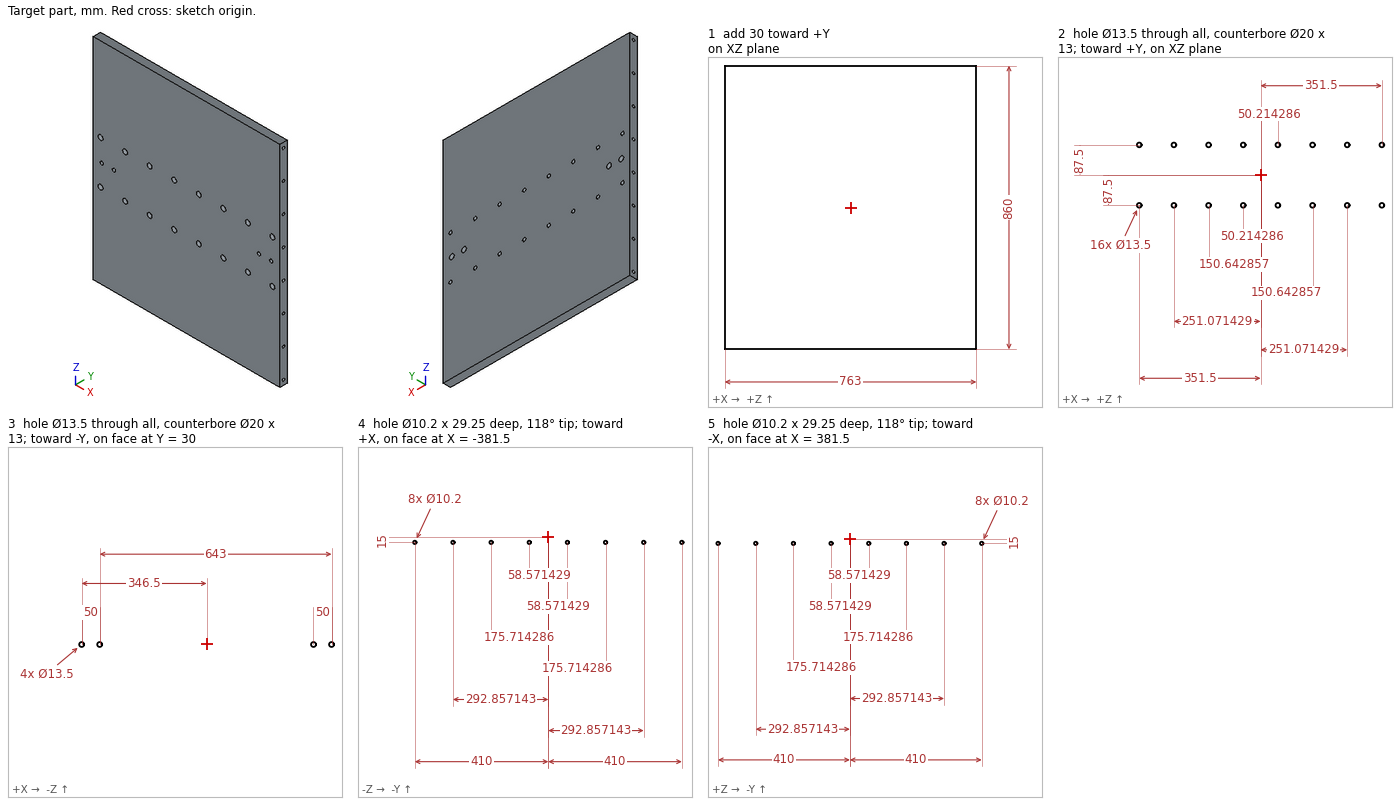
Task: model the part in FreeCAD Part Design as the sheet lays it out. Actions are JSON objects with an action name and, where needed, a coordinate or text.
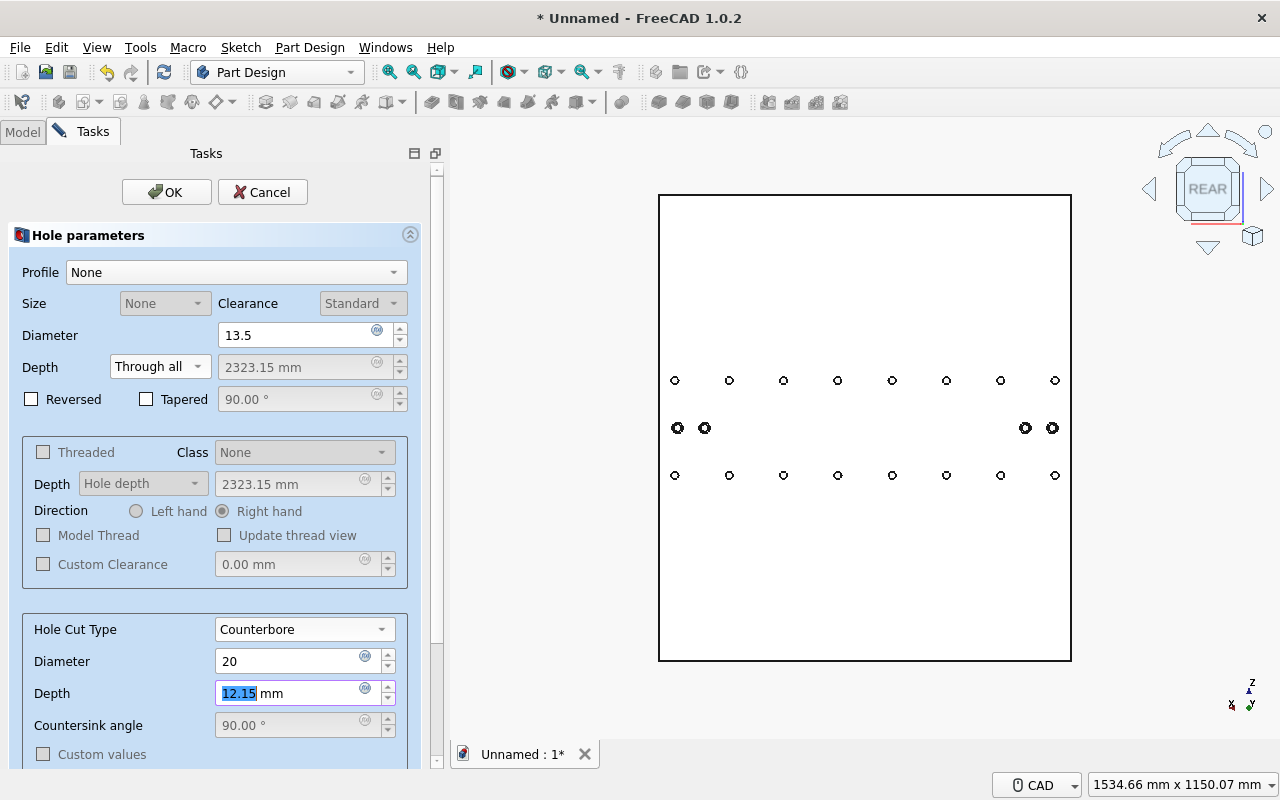
{"action": "type", "text": "13"}
{"action": "key", "text": "Tab"}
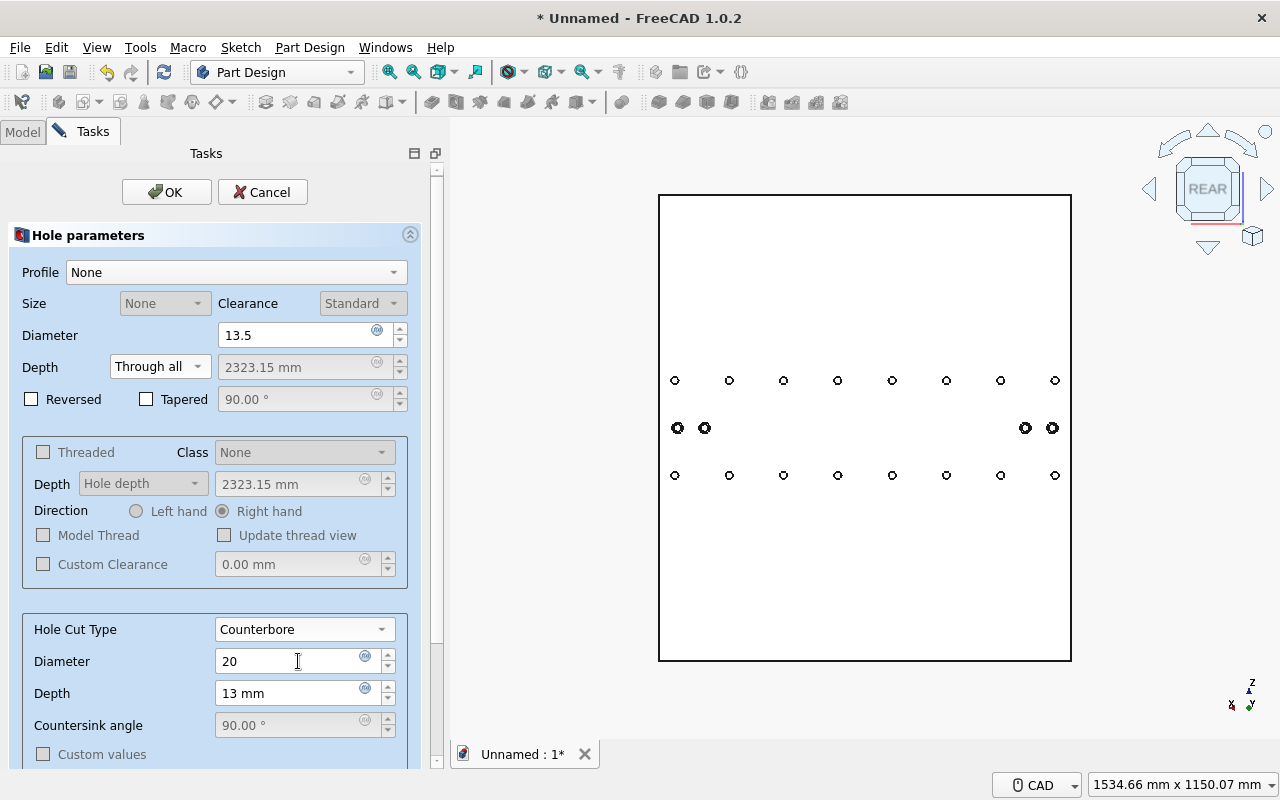
{"action": "left_click", "coordinate": [167, 192]}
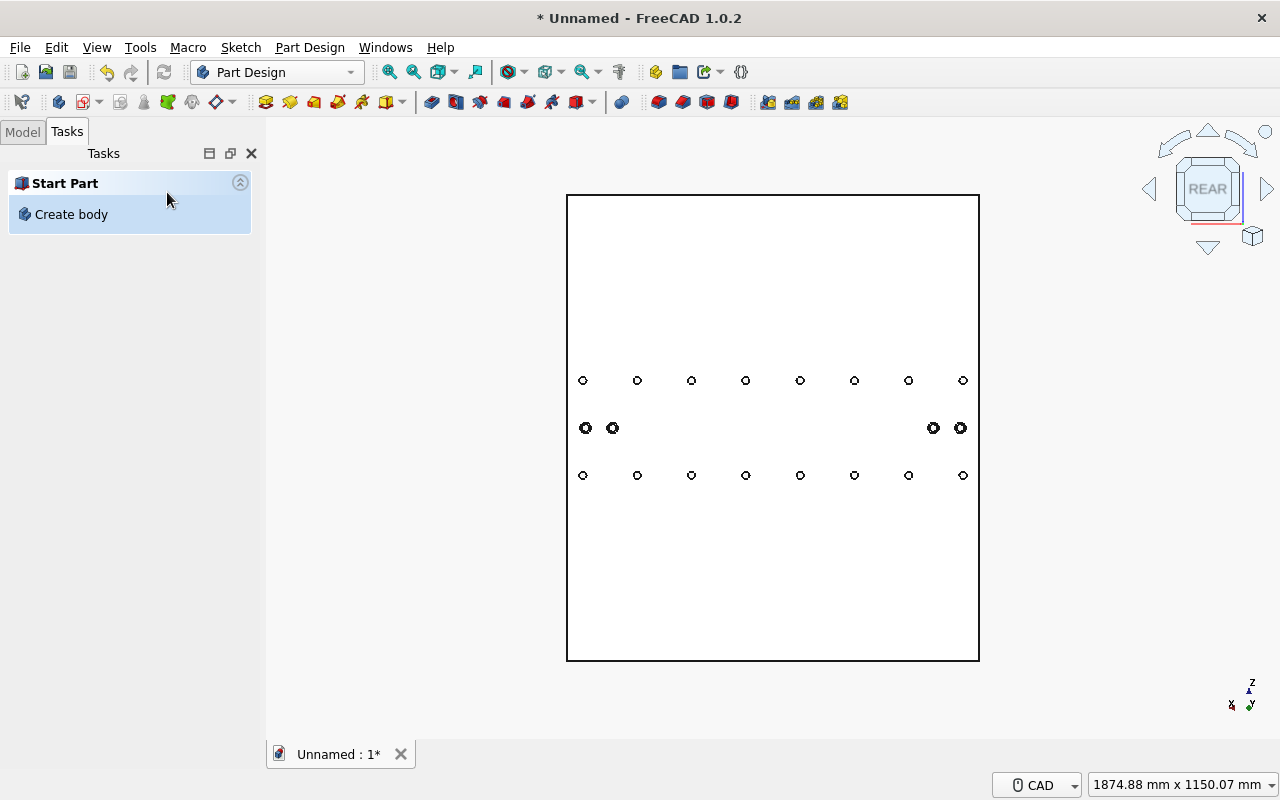
{"action": "key", "text": "6"}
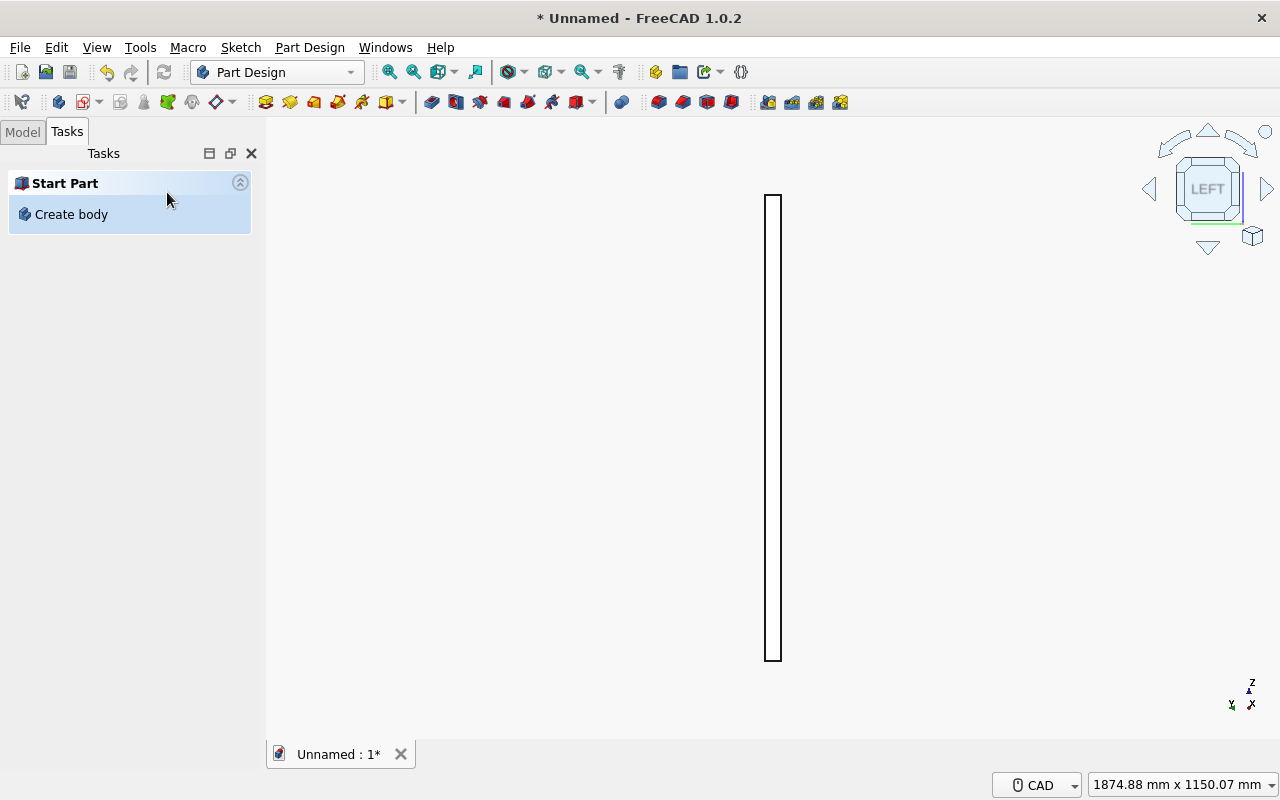
{"action": "left_click", "coordinate": [773, 228]}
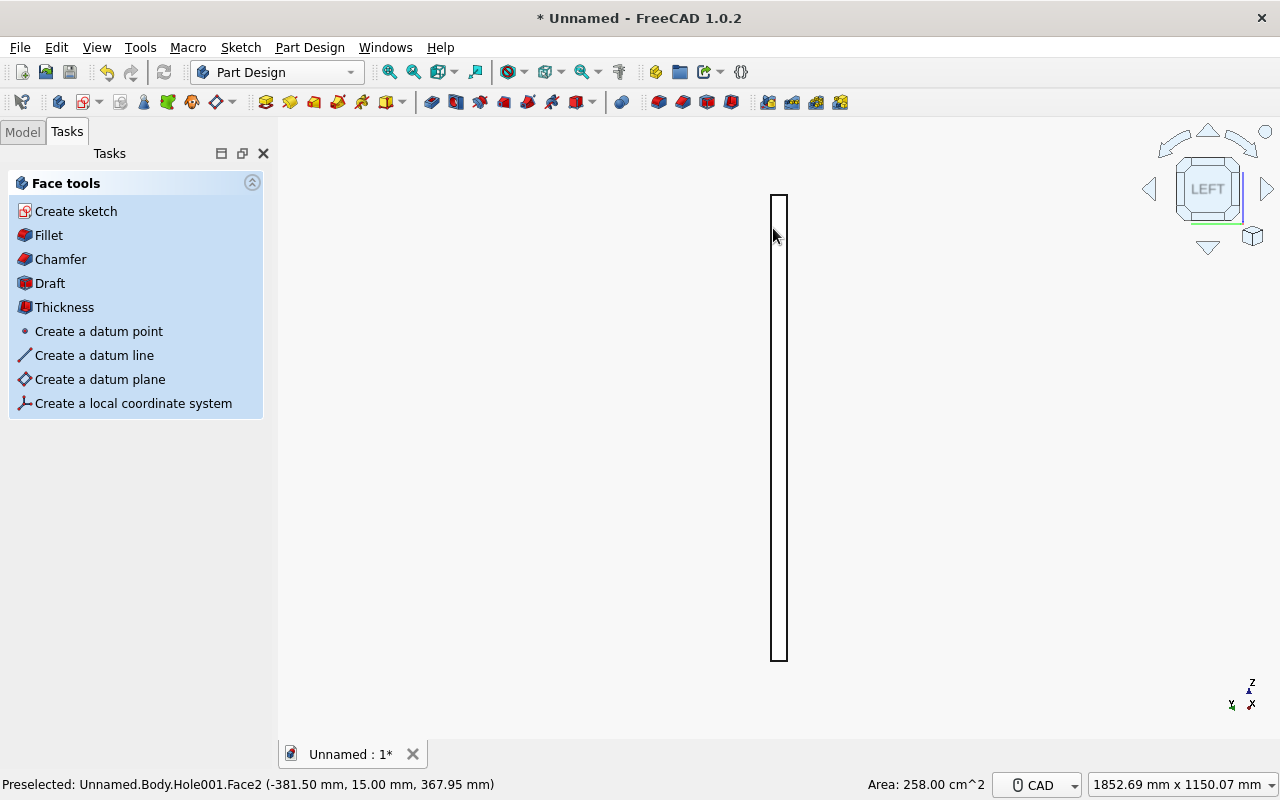
{"action": "left_click", "coordinate": [84, 102]}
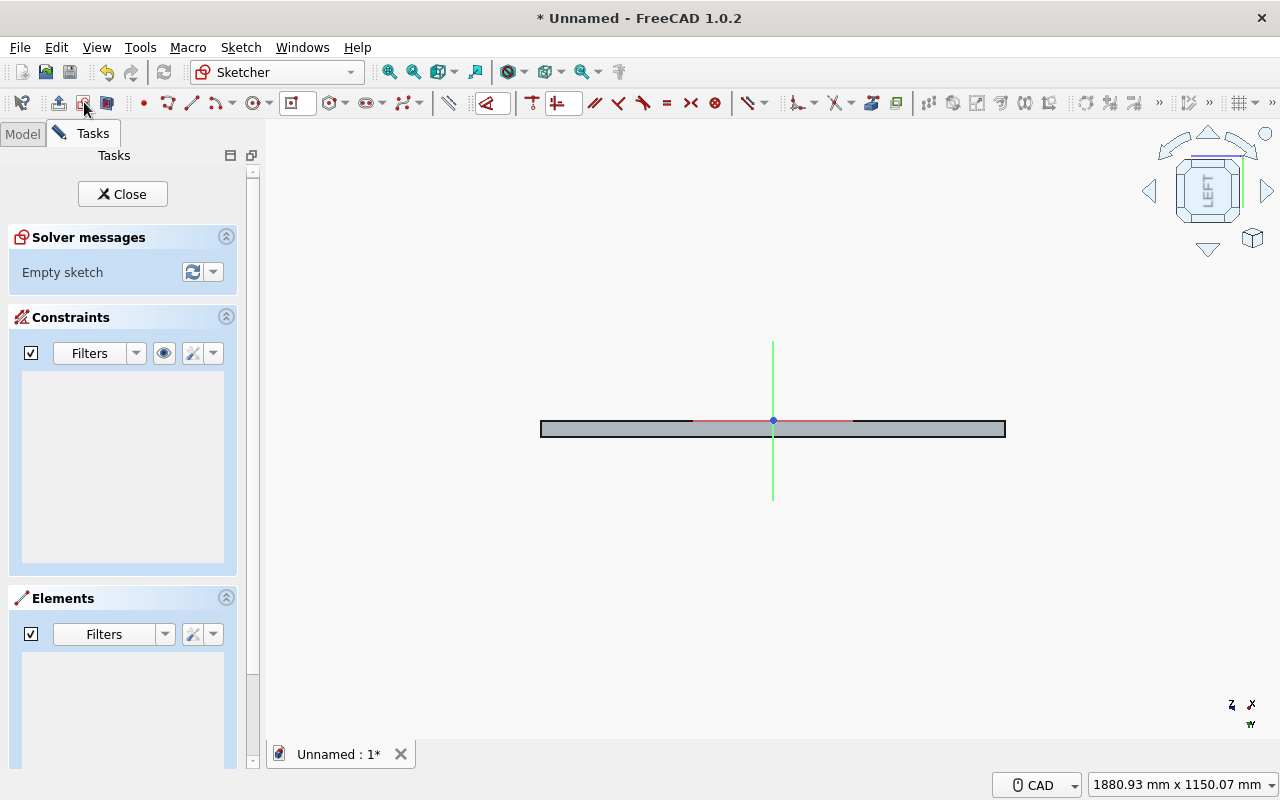
{"action": "left_click", "coordinate": [254, 104]}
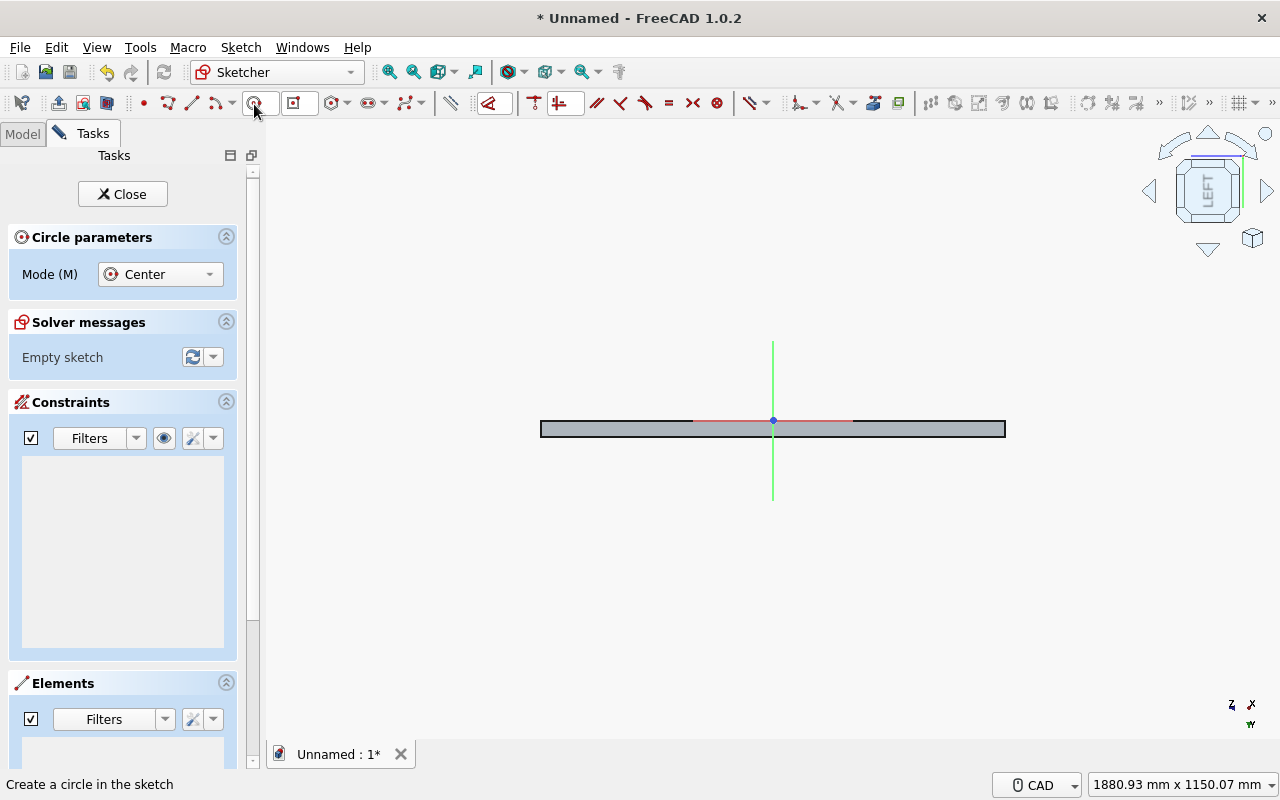
{"action": "scroll", "coordinate": [552, 429], "scroll_direction": "up", "scroll_amount": 11}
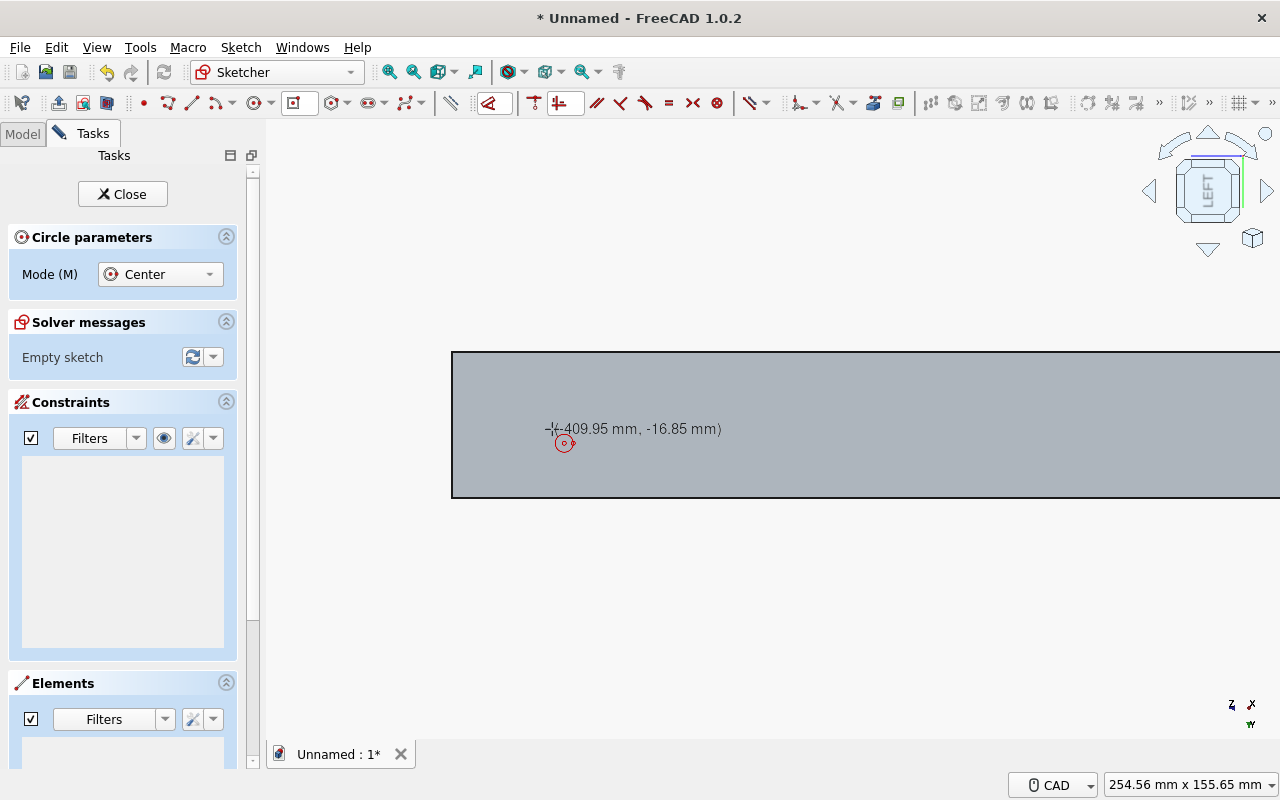
{"action": "scroll", "coordinate": [417, 433], "scroll_direction": "down", "scroll_amount": 10}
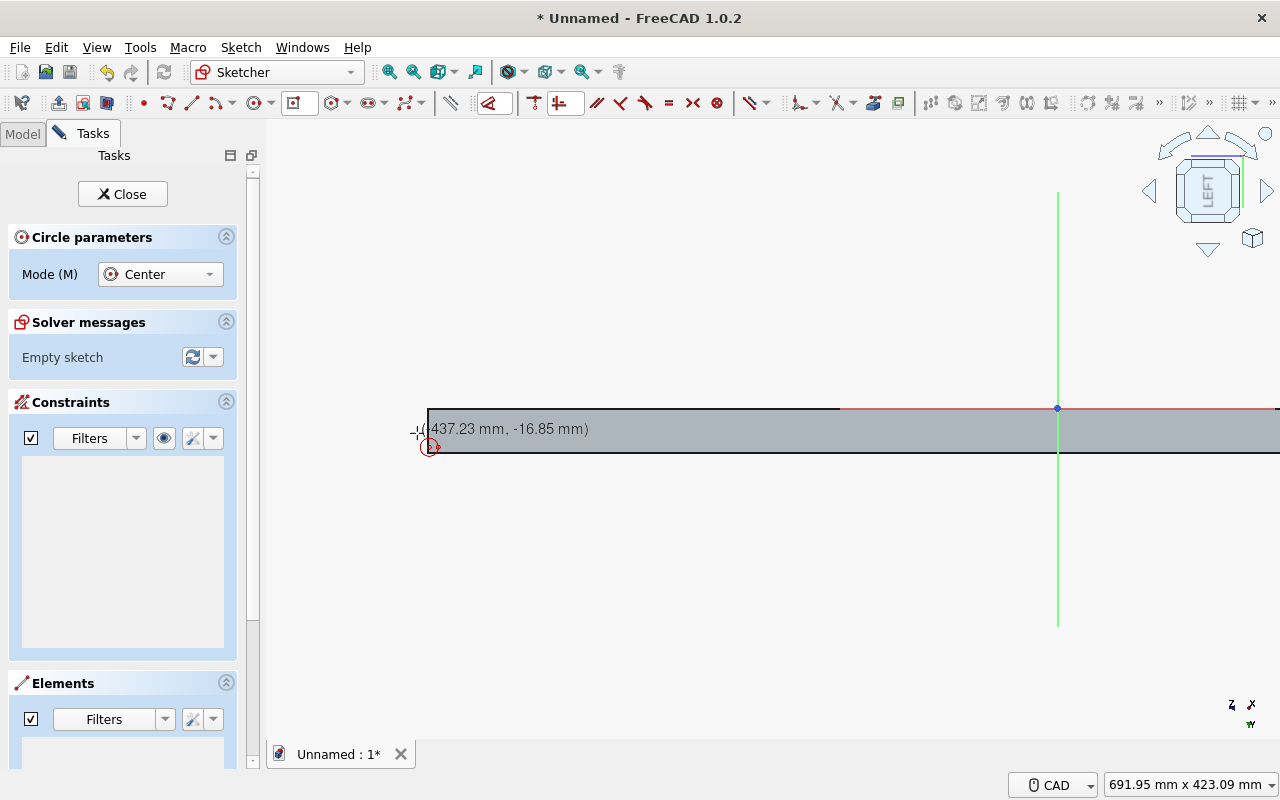
{"action": "scroll", "coordinate": [435, 432], "scroll_direction": "up", "scroll_amount": 3}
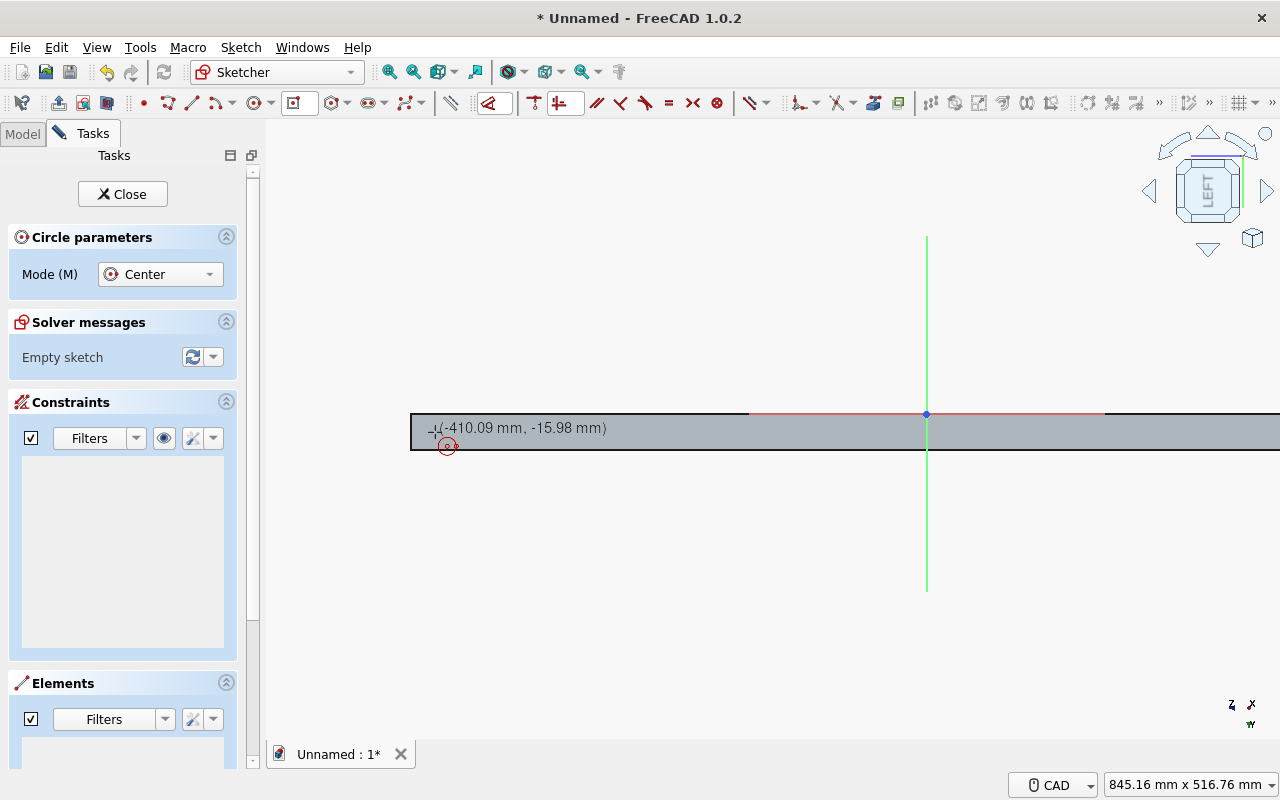
{"action": "left_click", "coordinate": [435, 432]}